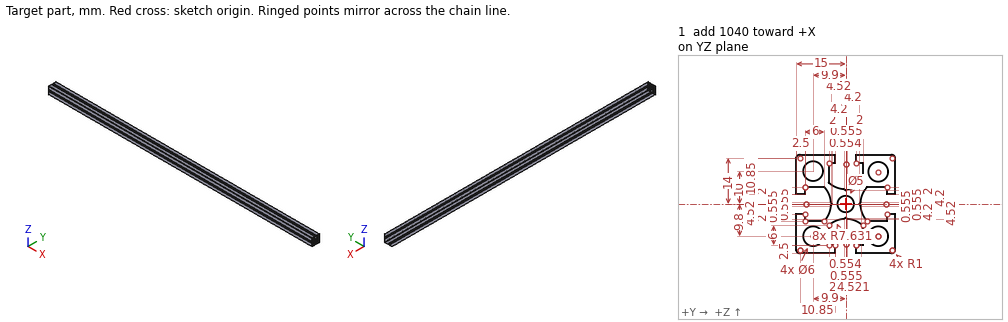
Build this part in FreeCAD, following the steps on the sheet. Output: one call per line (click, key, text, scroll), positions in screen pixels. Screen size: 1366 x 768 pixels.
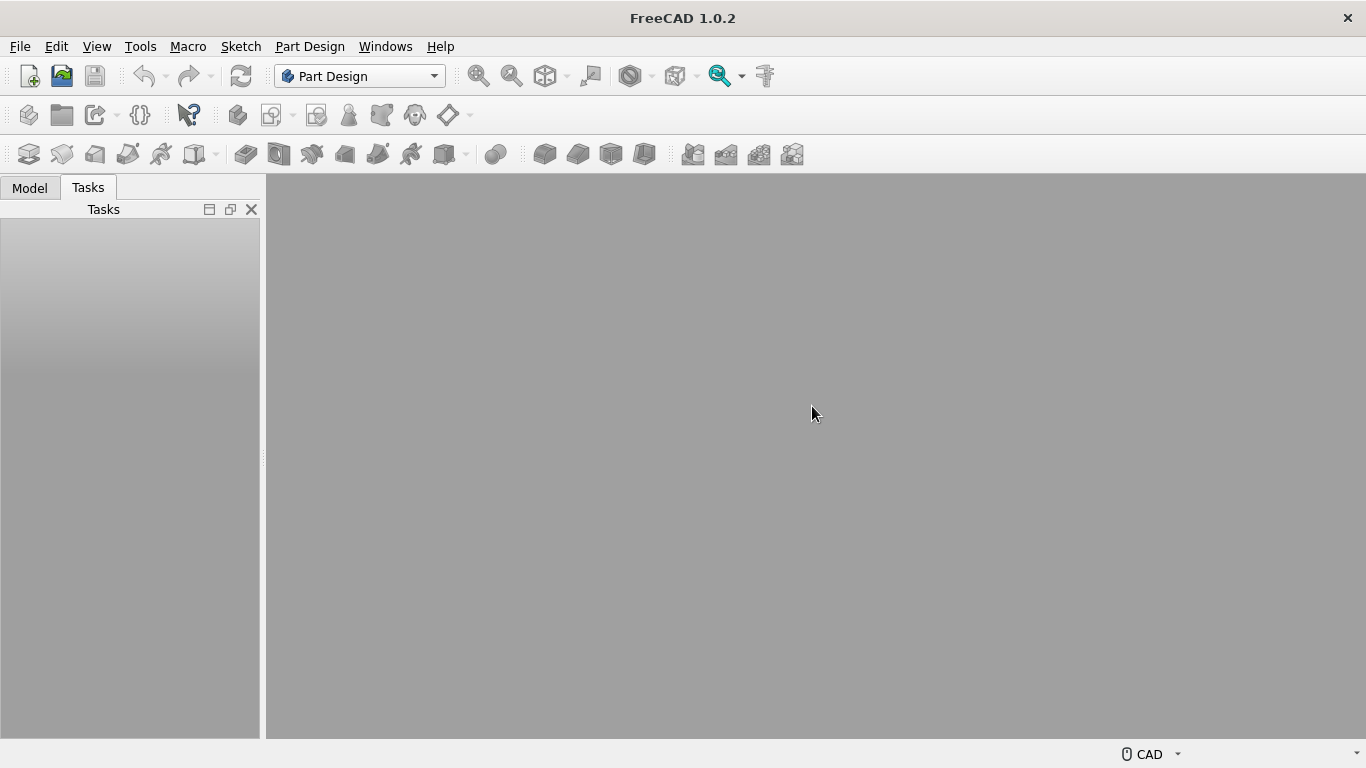
key(ctrl+n)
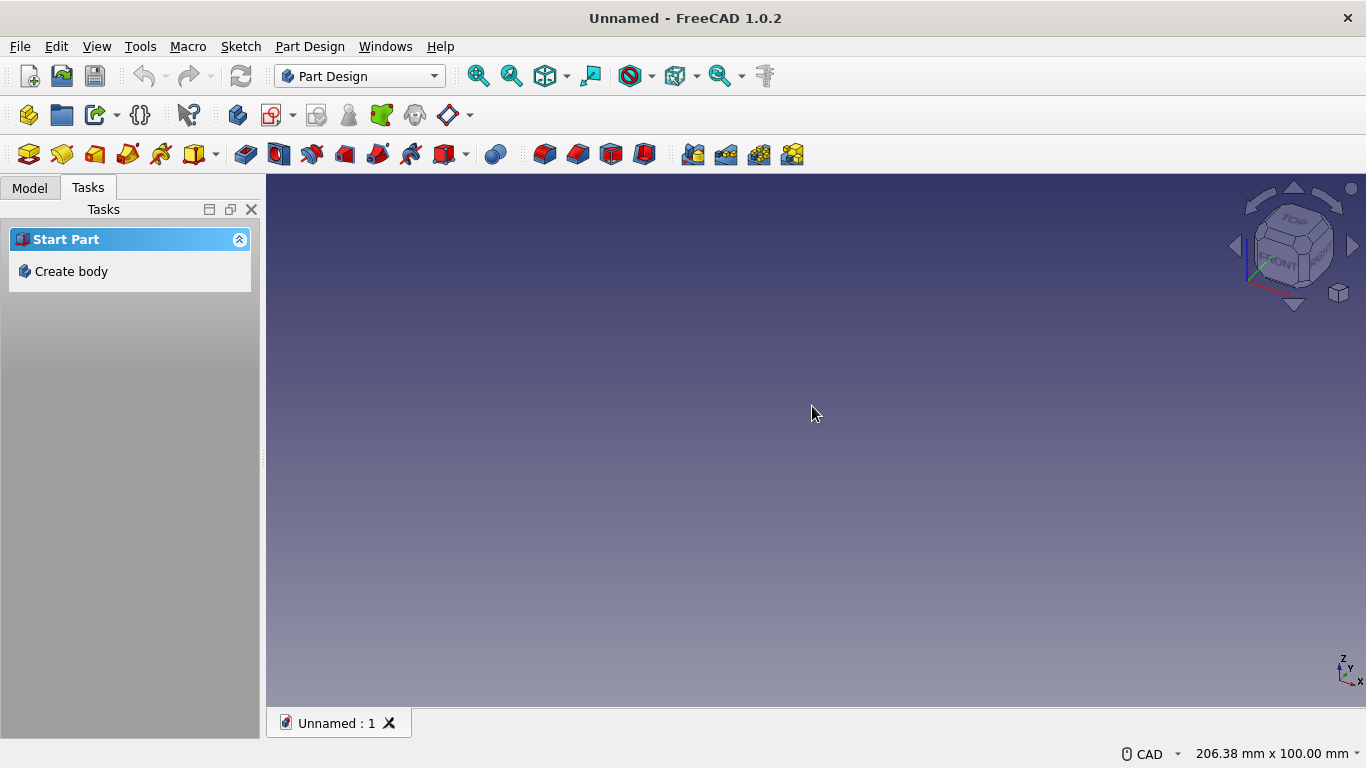
click(270, 116)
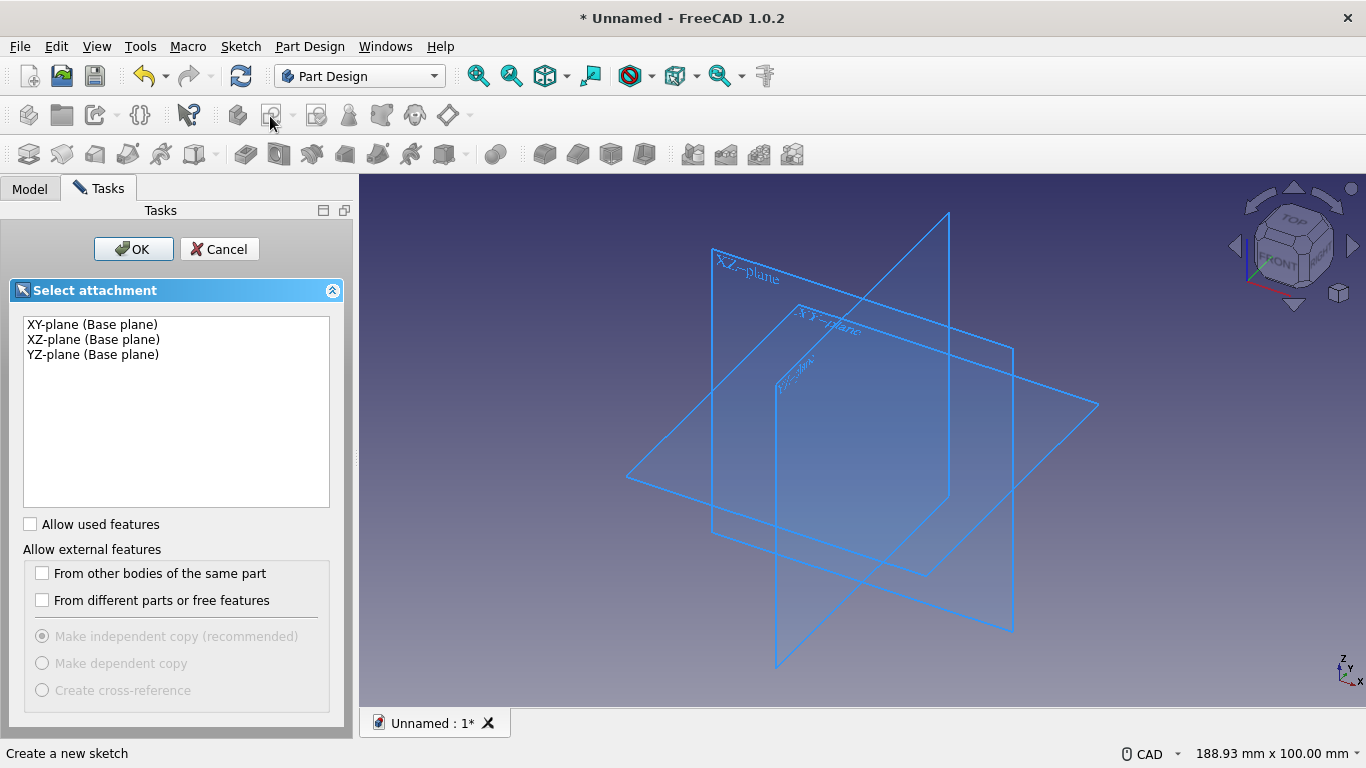
click(84, 354)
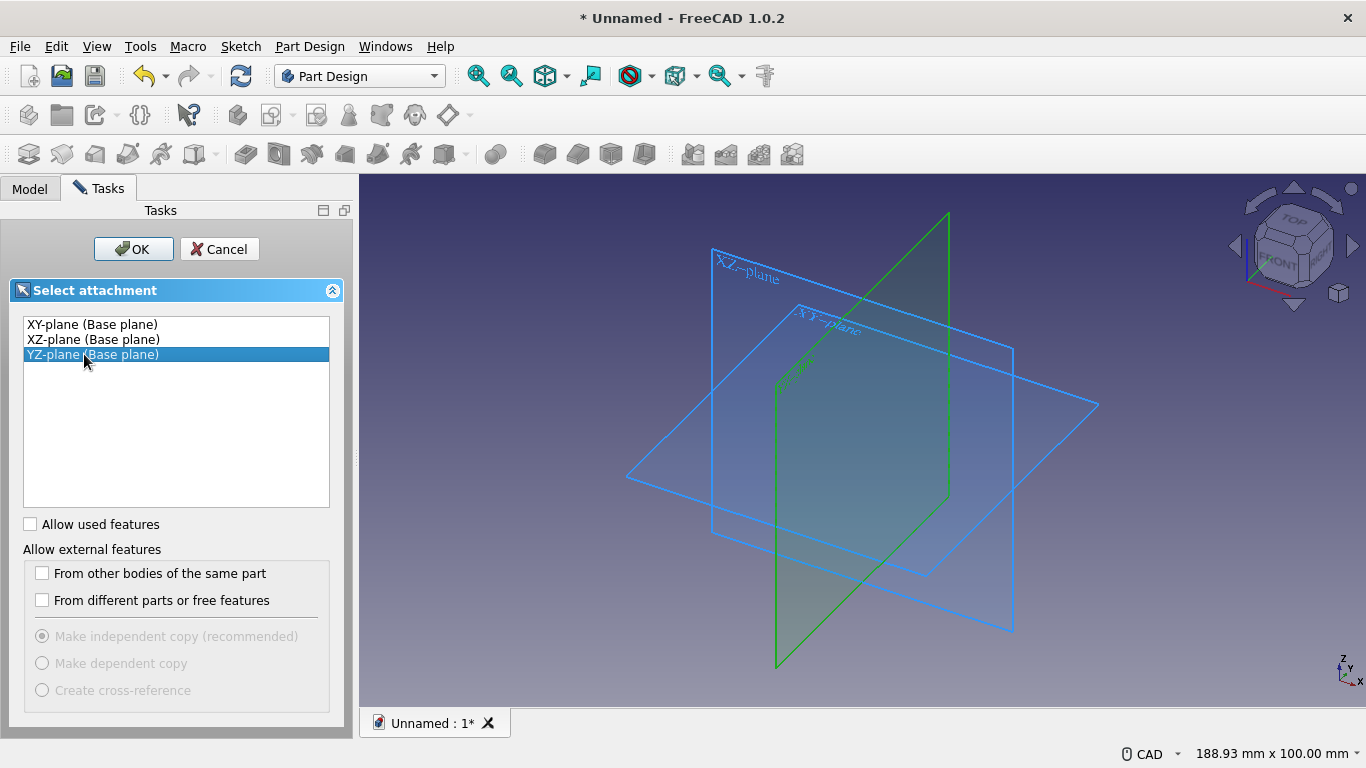
click(134, 249)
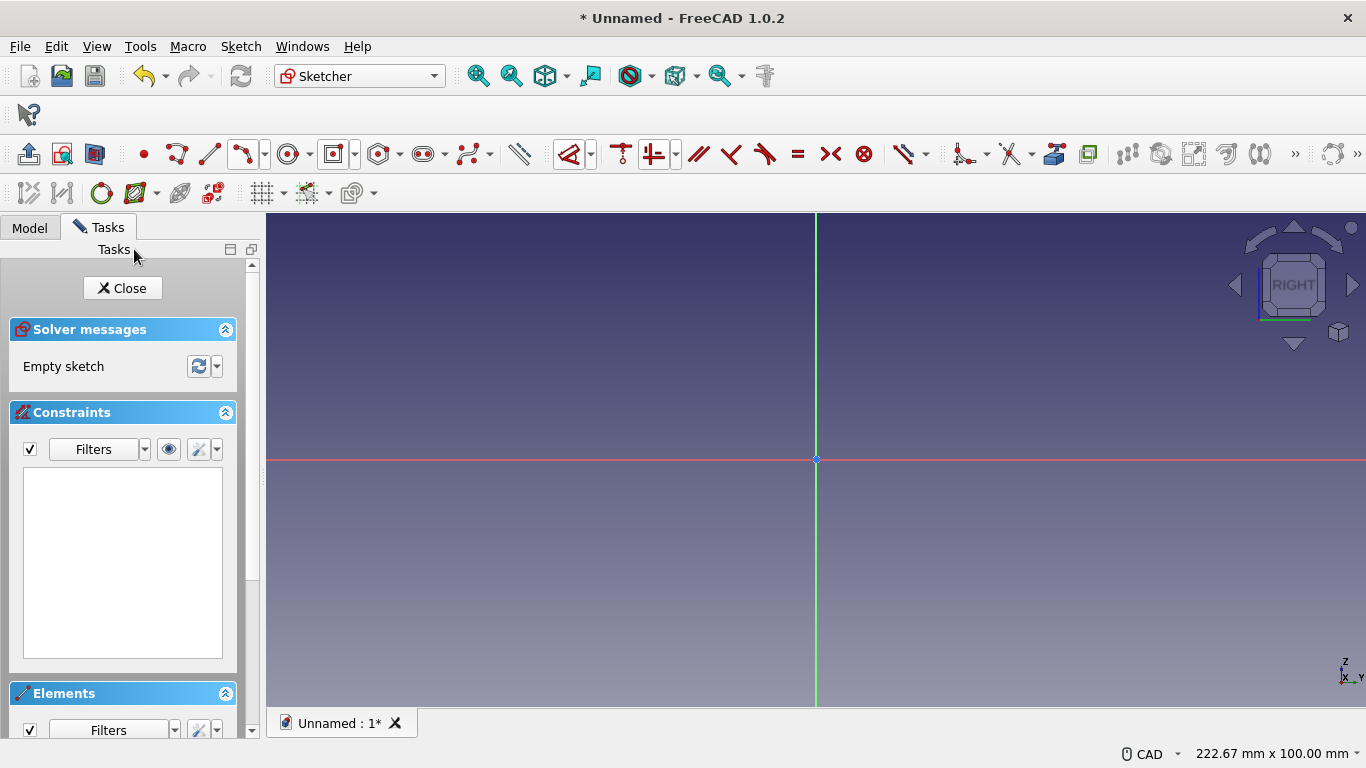
scroll(872, 460, up, 4)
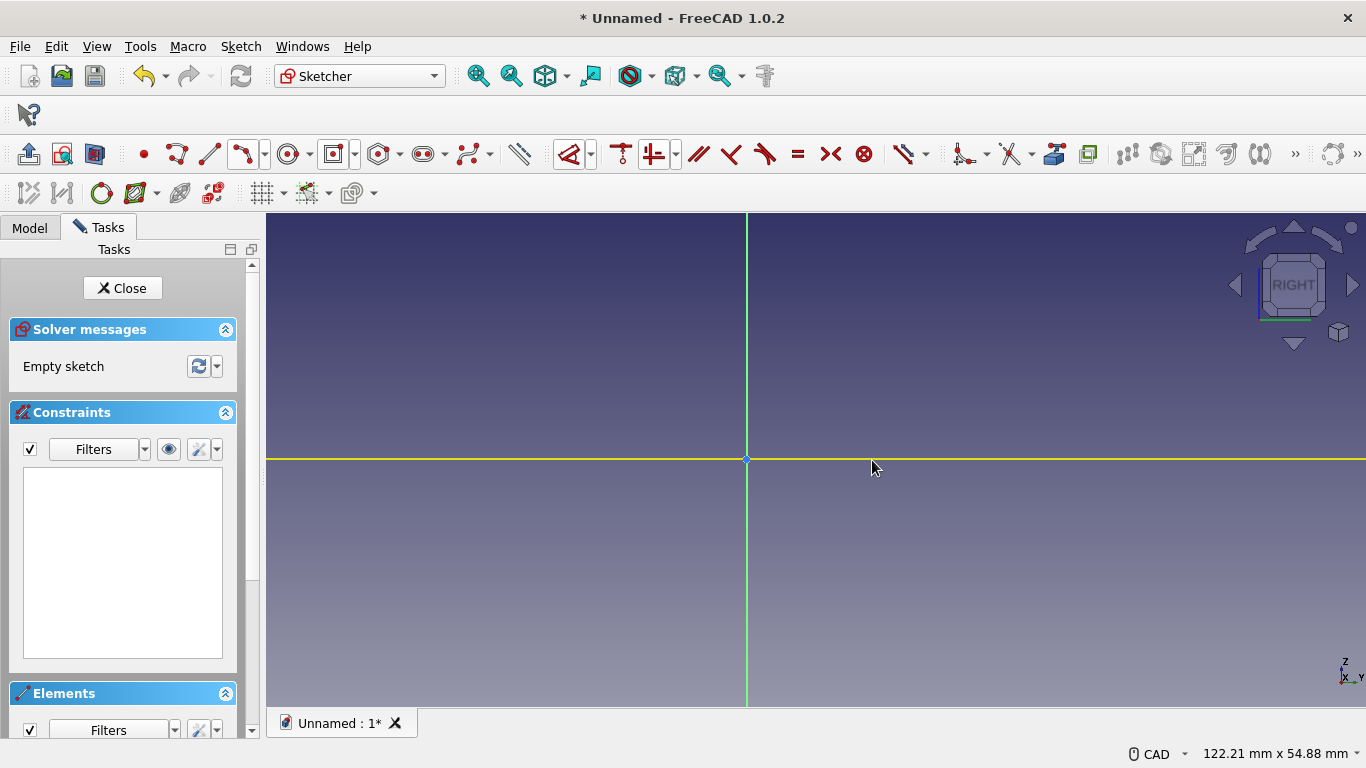
key(g)
key(m)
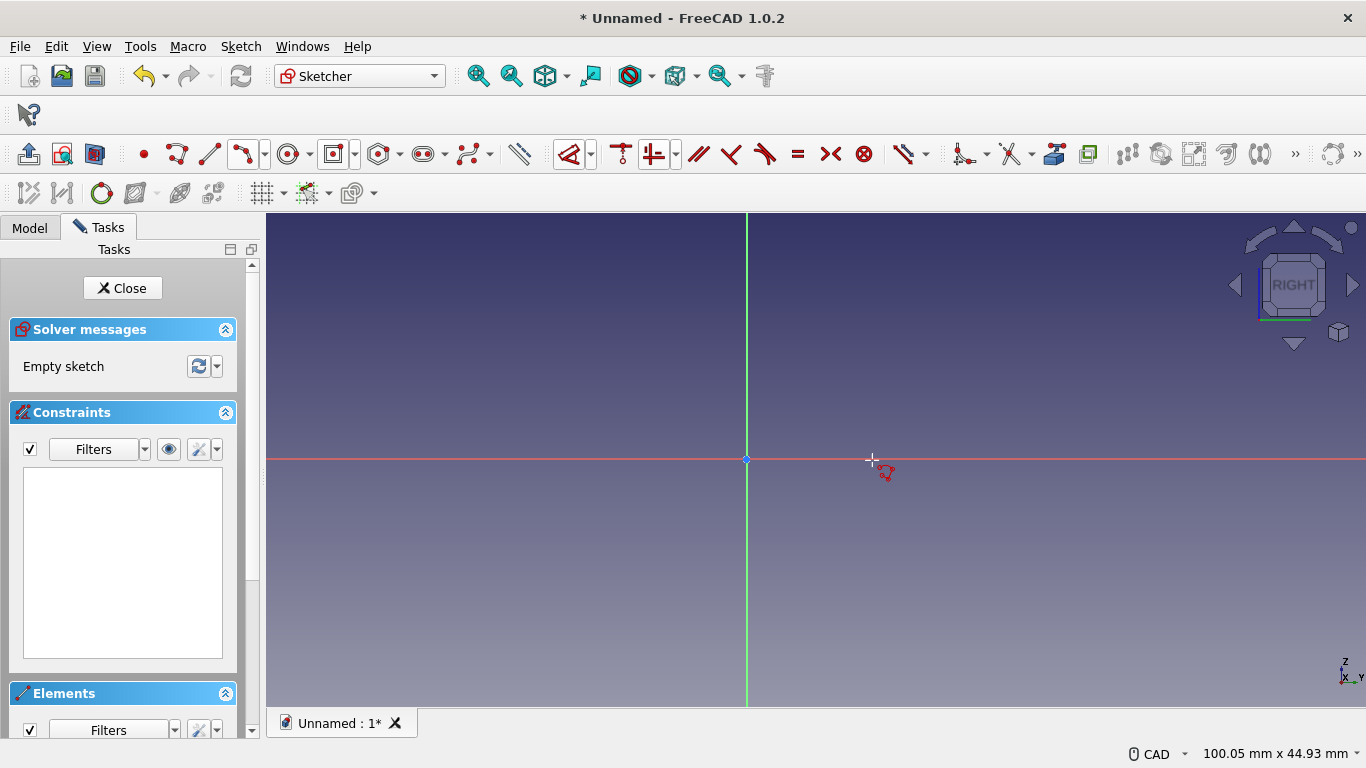
click(582, 305)
click(582, 425)
click(609, 425)
click(609, 403)
click(675, 403)
right_click(675, 403)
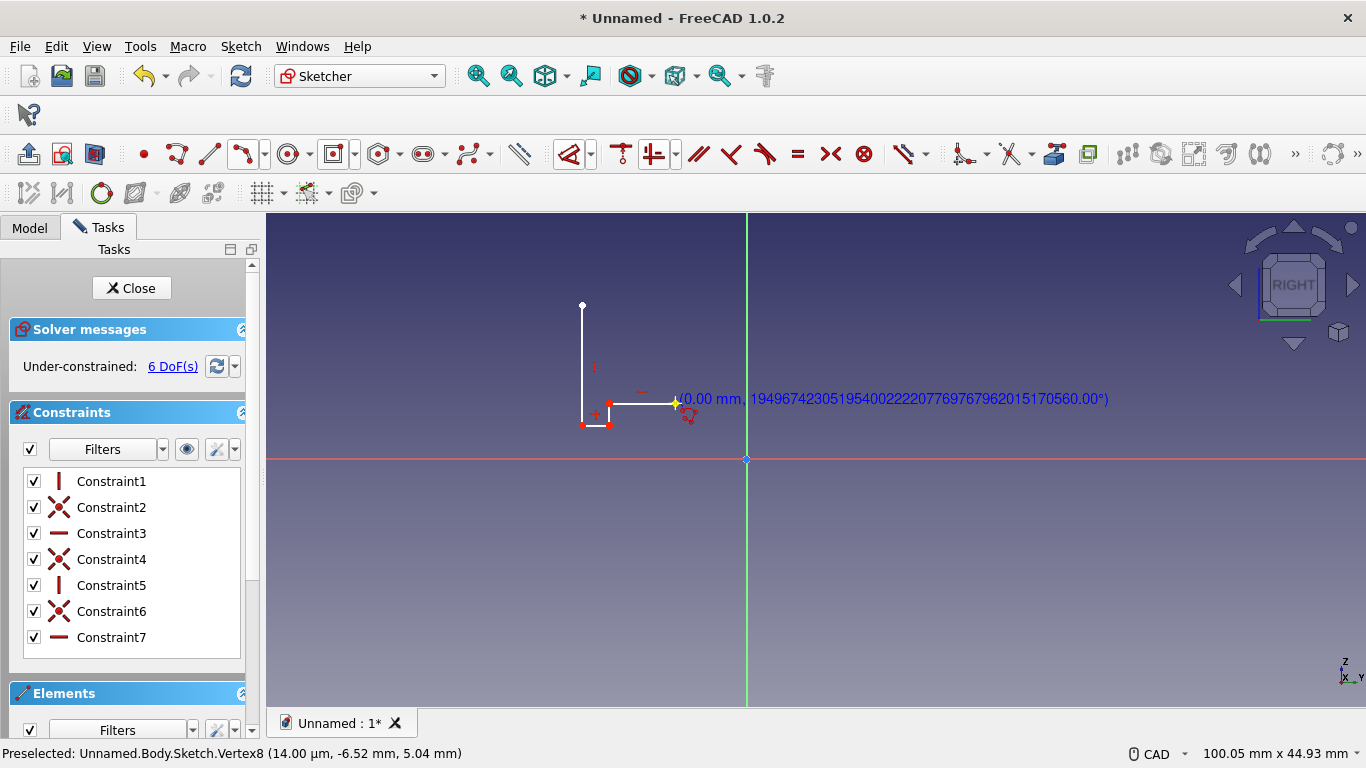
scroll(697, 453, up, 5)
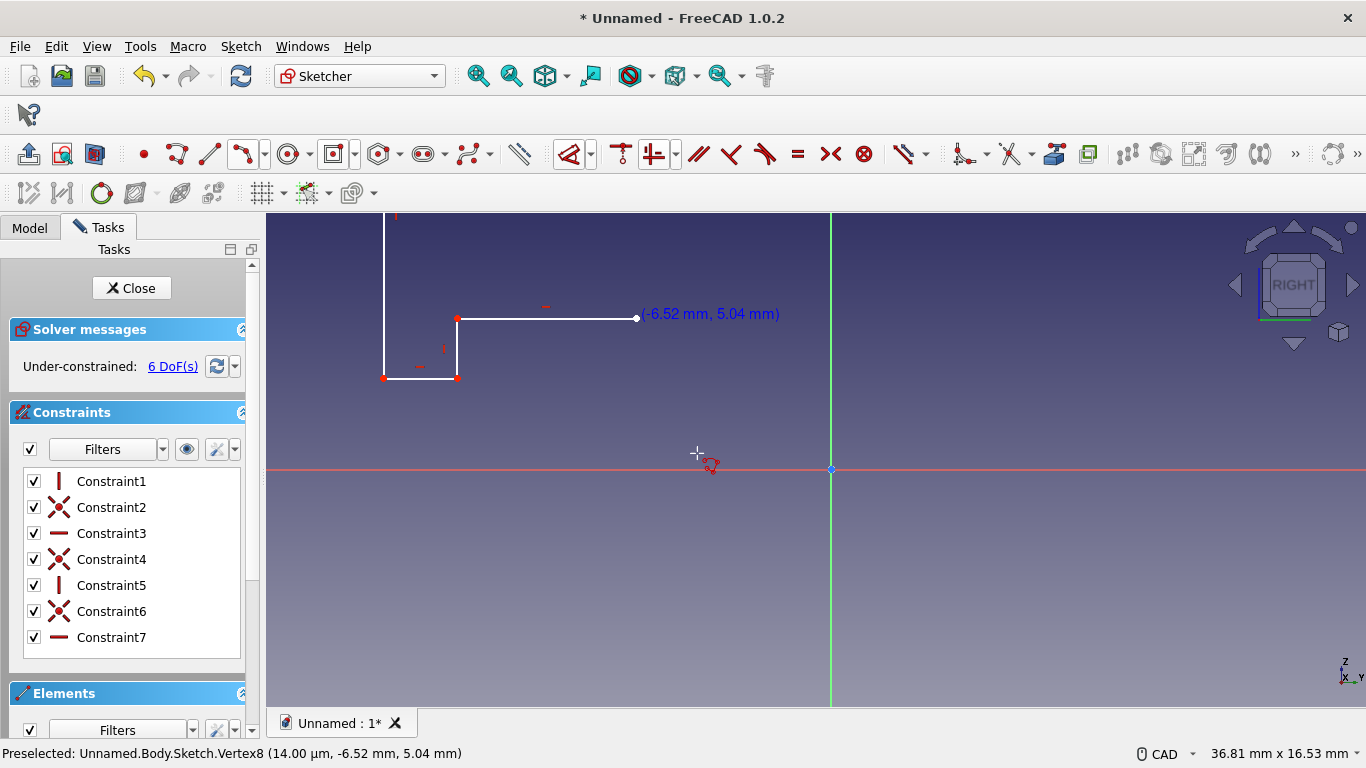
click(696, 453)
click(706, 470)
click(696, 486)
right_click(696, 486)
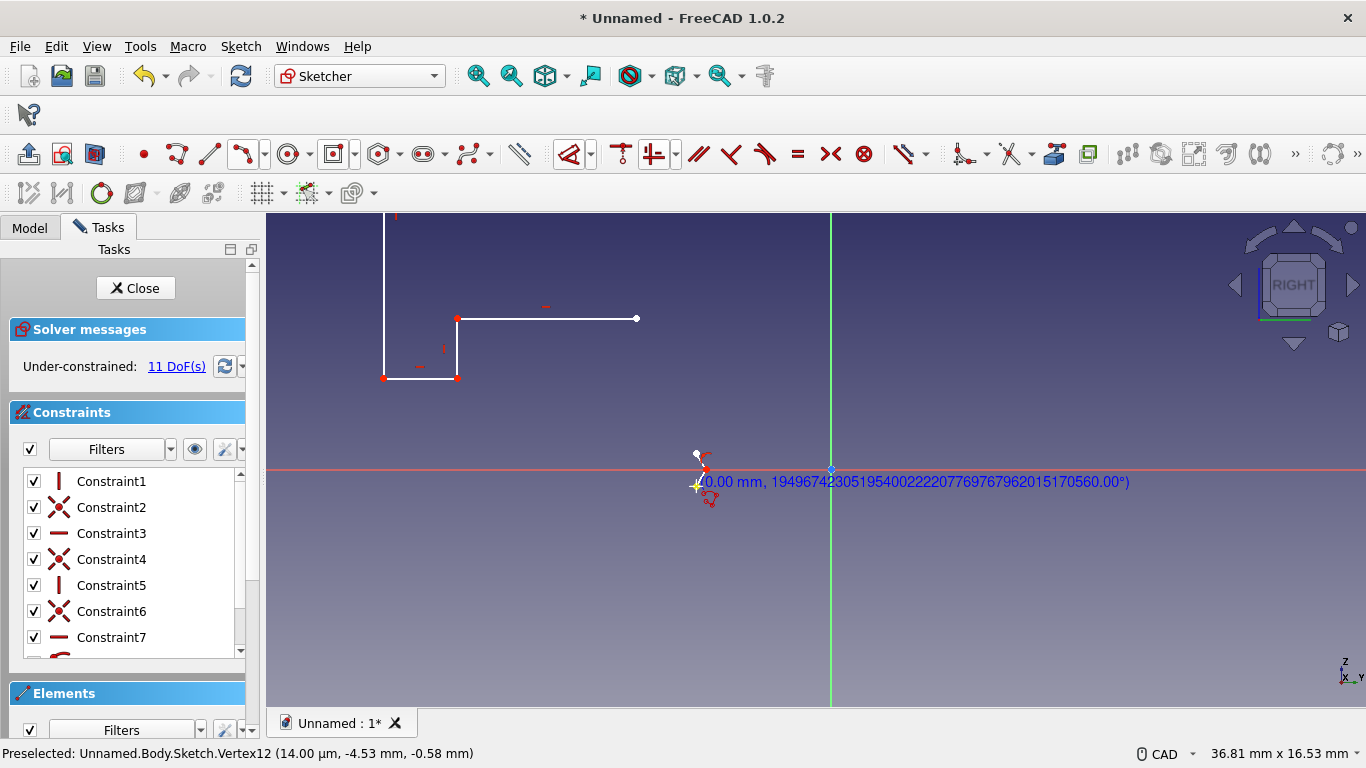
click(637, 623)
click(458, 623)
click(458, 564)
click(383, 564)